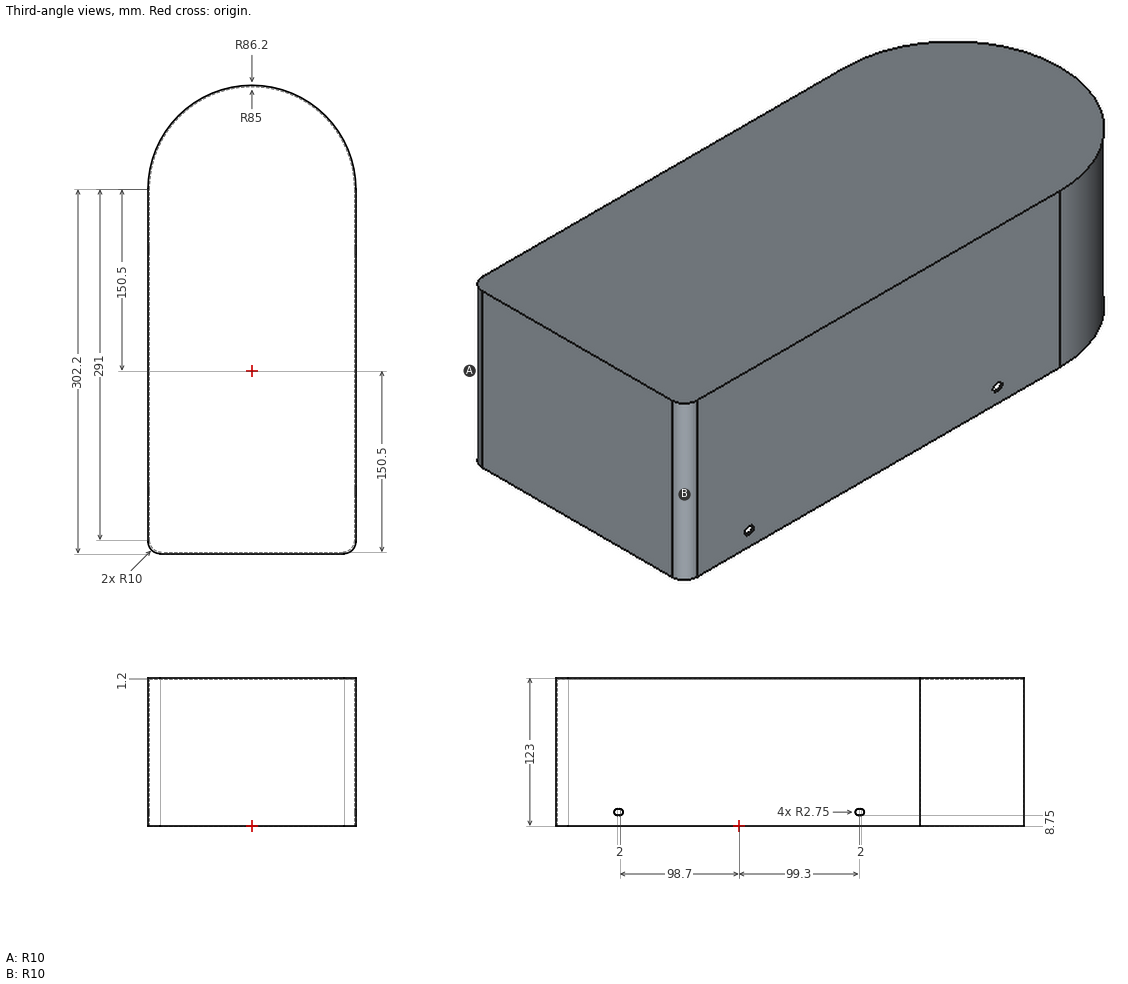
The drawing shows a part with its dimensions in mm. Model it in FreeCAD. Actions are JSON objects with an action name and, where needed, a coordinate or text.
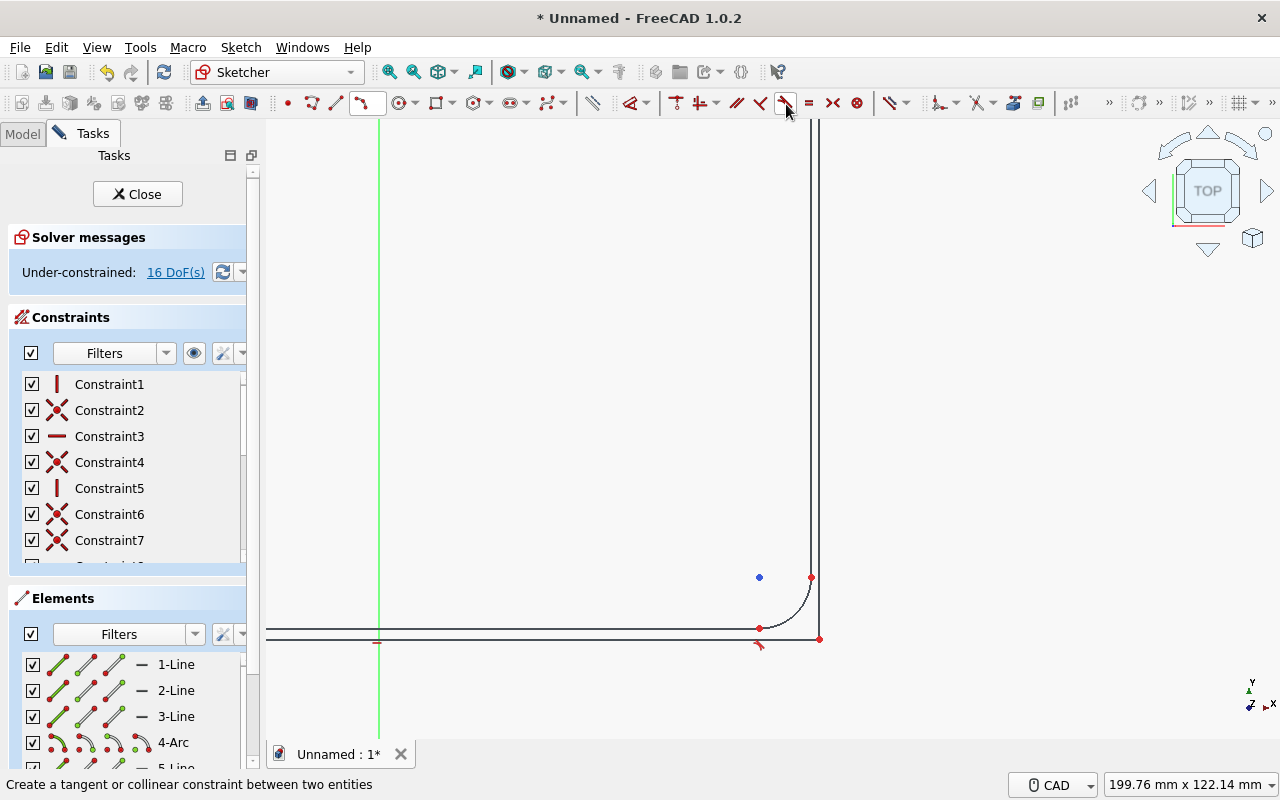
{"action": "scroll", "coordinate": [787, 626], "scroll_direction": "down", "scroll_amount": 8}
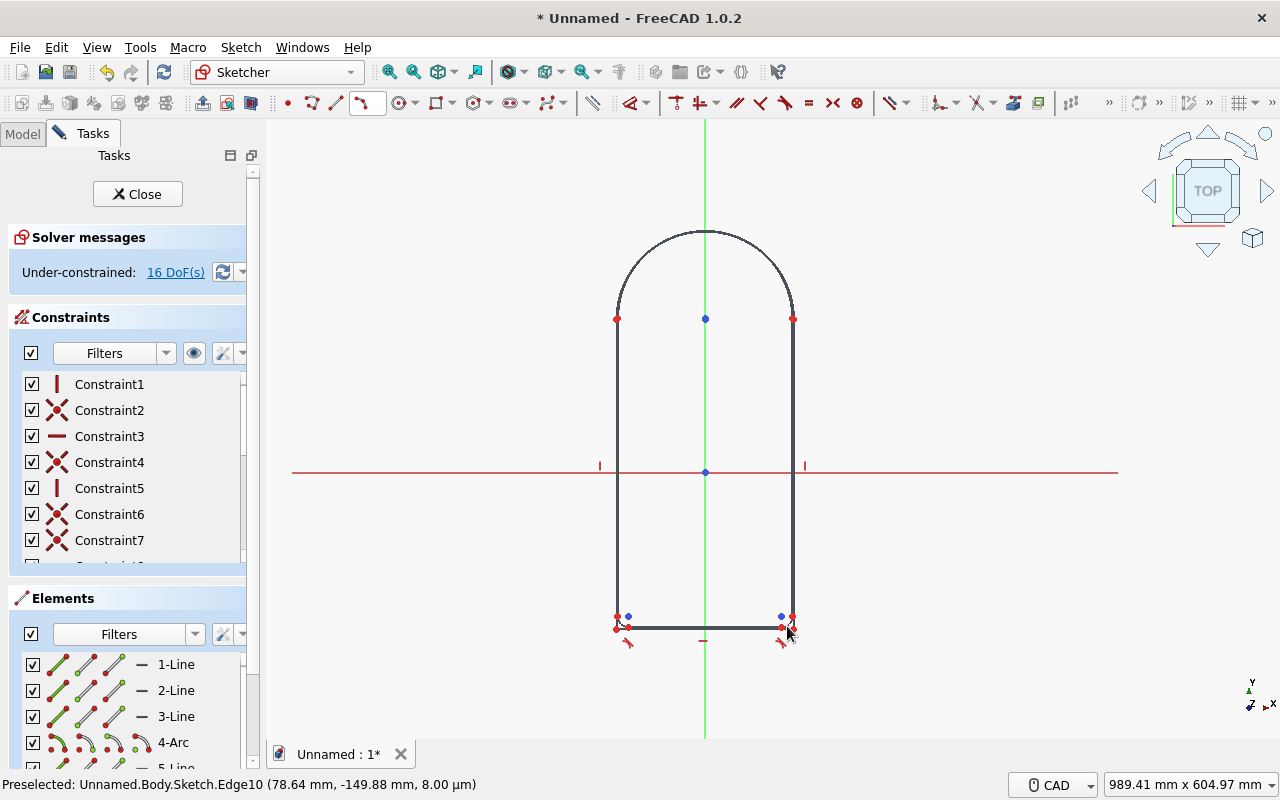
{"action": "scroll", "coordinate": [618, 527], "scroll_direction": "up", "scroll_amount": 12}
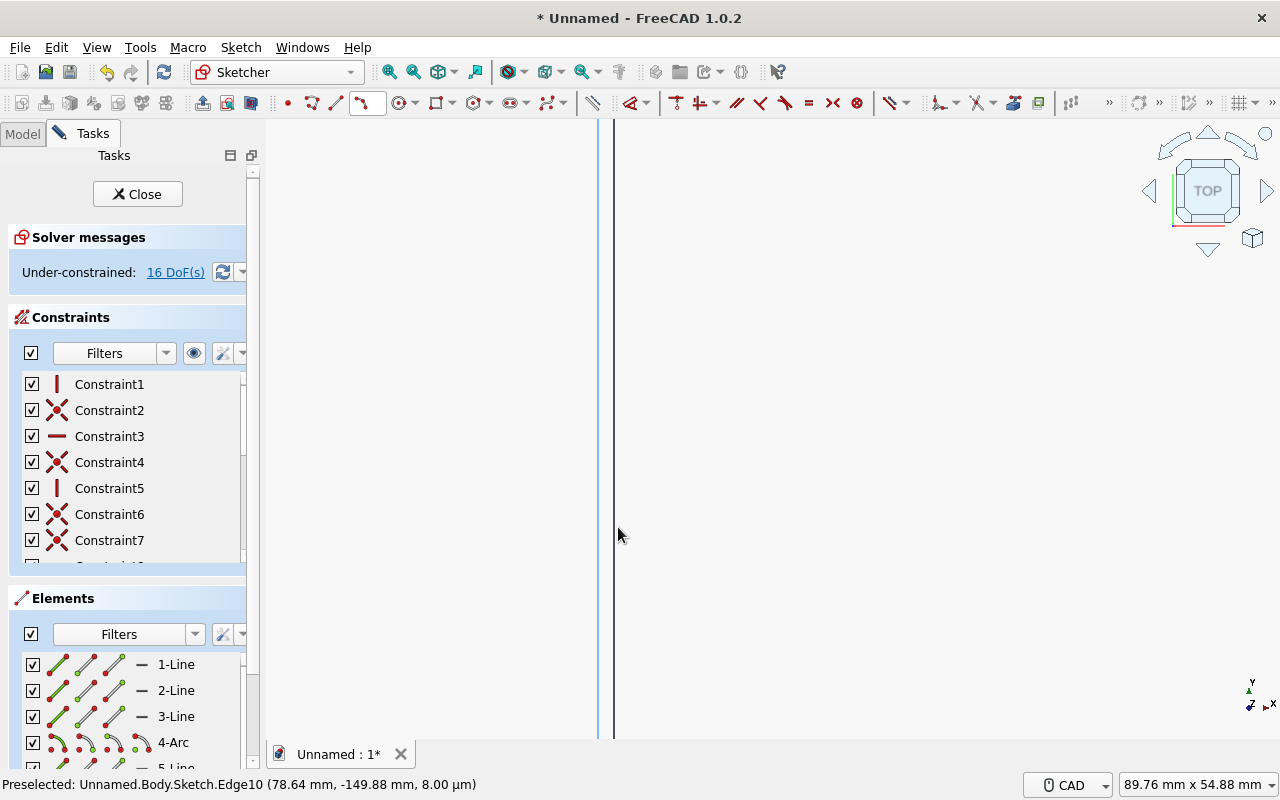
{"action": "left_click", "coordinate": [614, 525]}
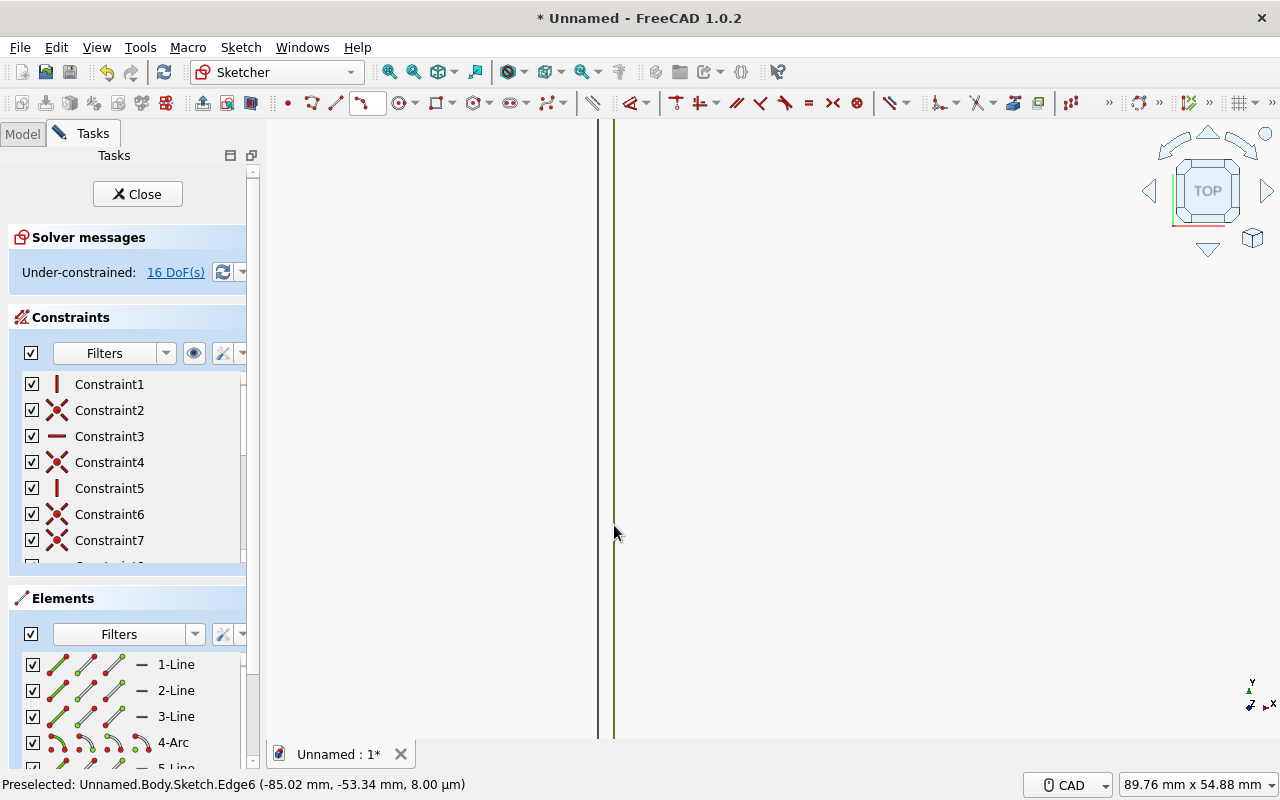
{"action": "scroll", "coordinate": [618, 527], "scroll_direction": "down", "scroll_amount": 12}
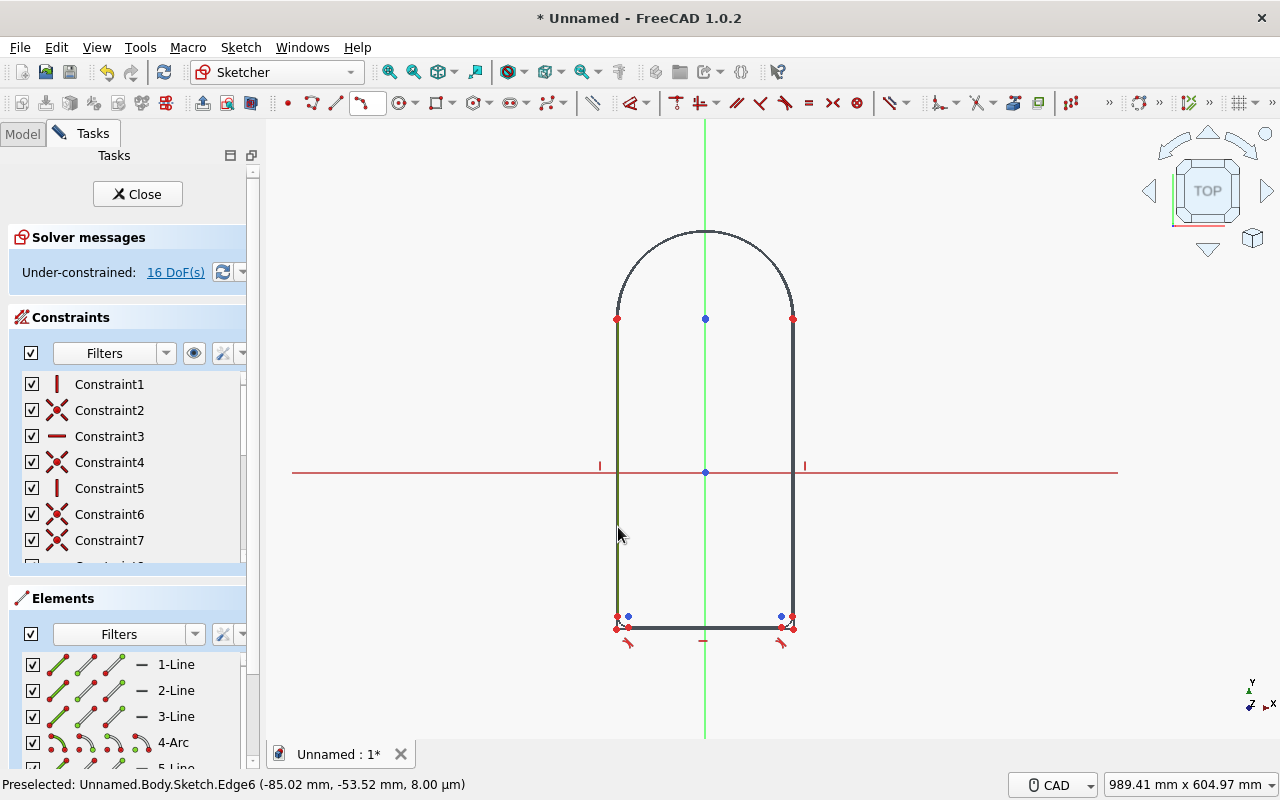
{"action": "scroll", "coordinate": [619, 622], "scroll_direction": "up", "scroll_amount": 9}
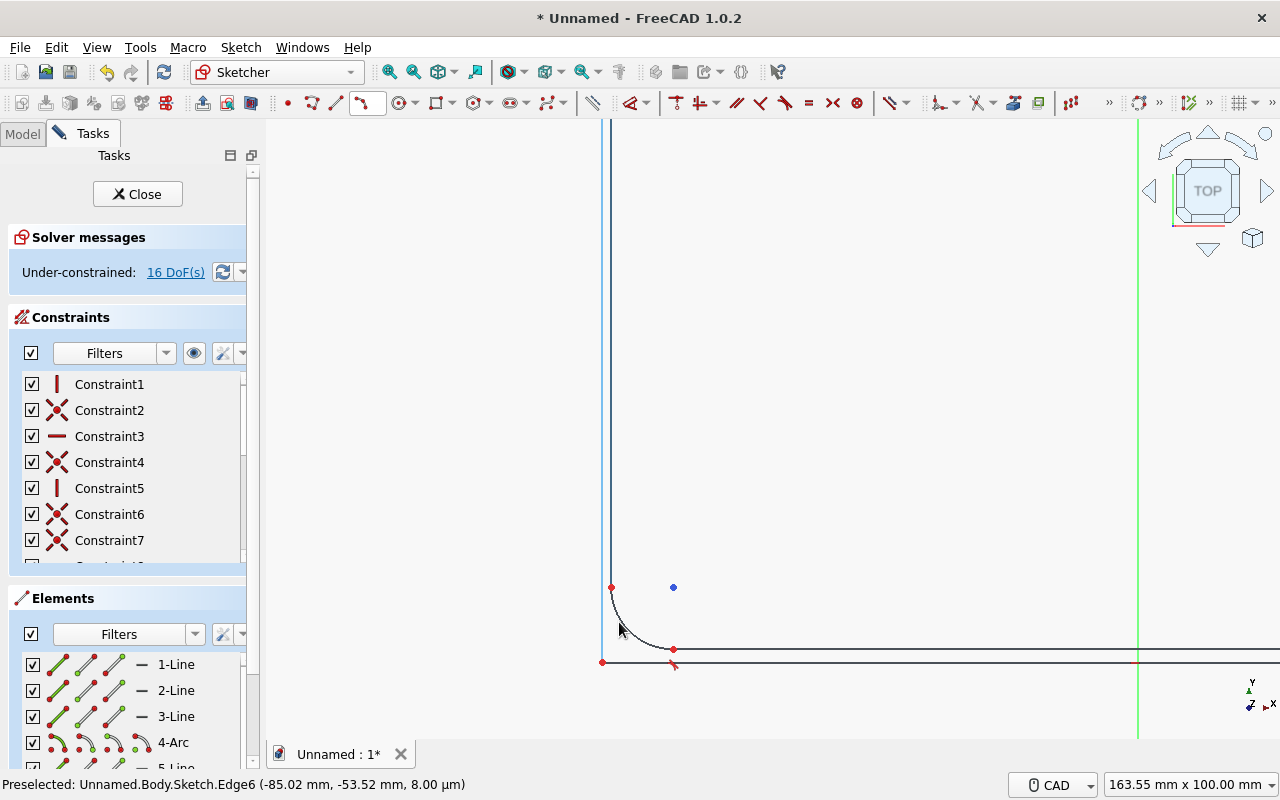
{"action": "left_click", "coordinate": [618, 615]}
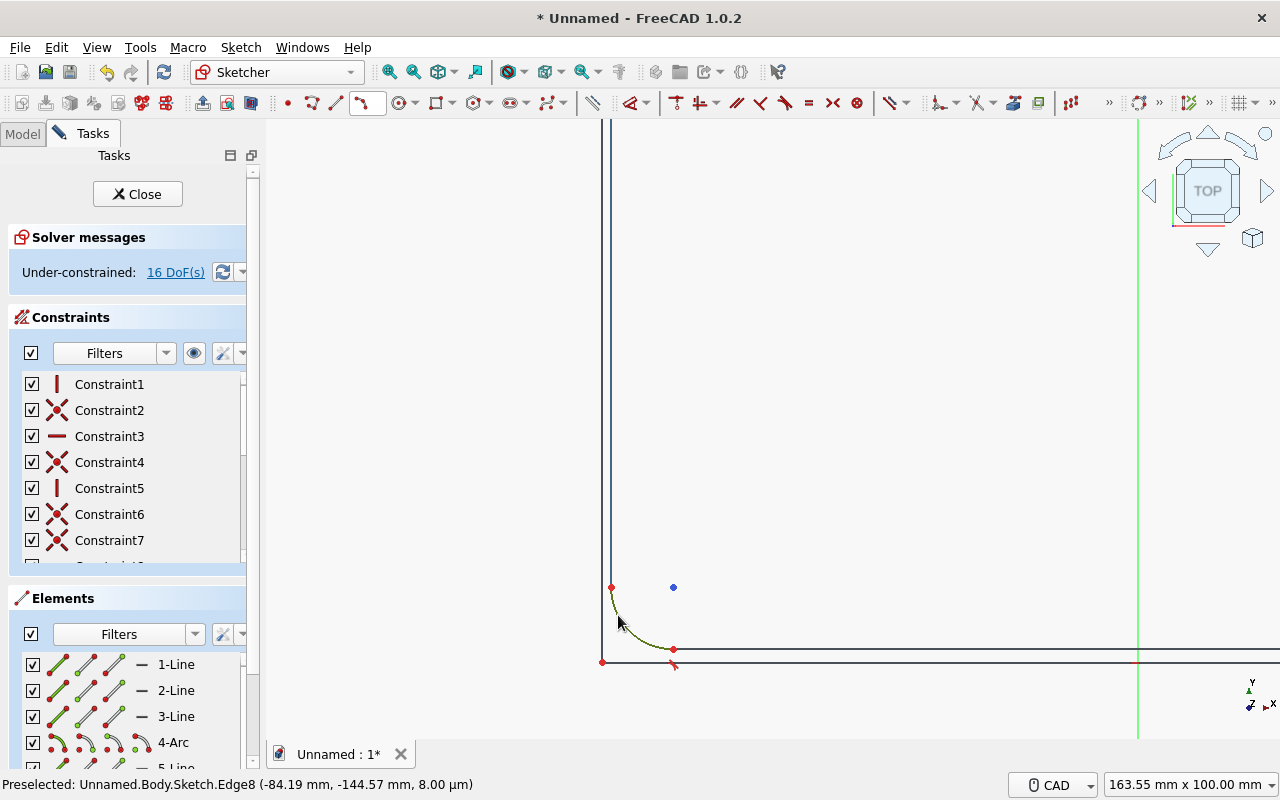
{"action": "key", "text": "t"}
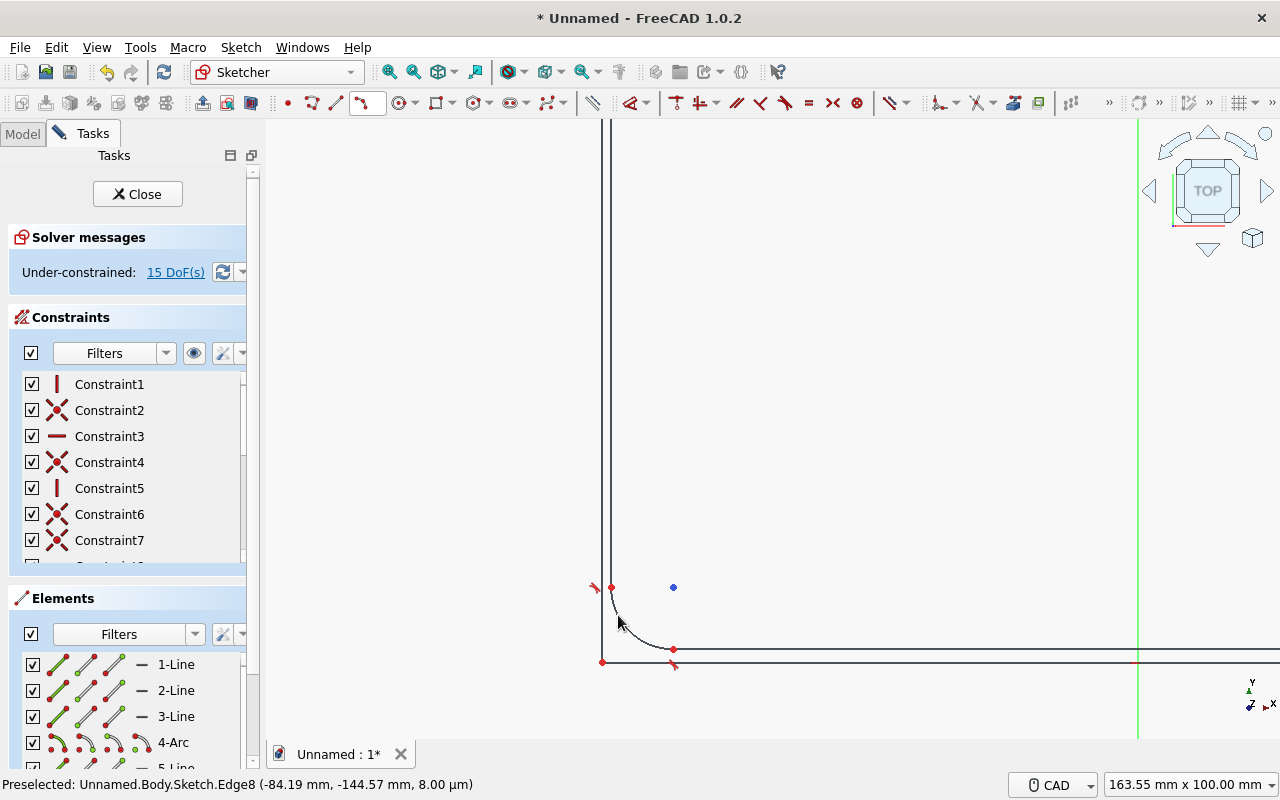
{"action": "scroll", "coordinate": [619, 622], "scroll_direction": "down", "scroll_amount": 9}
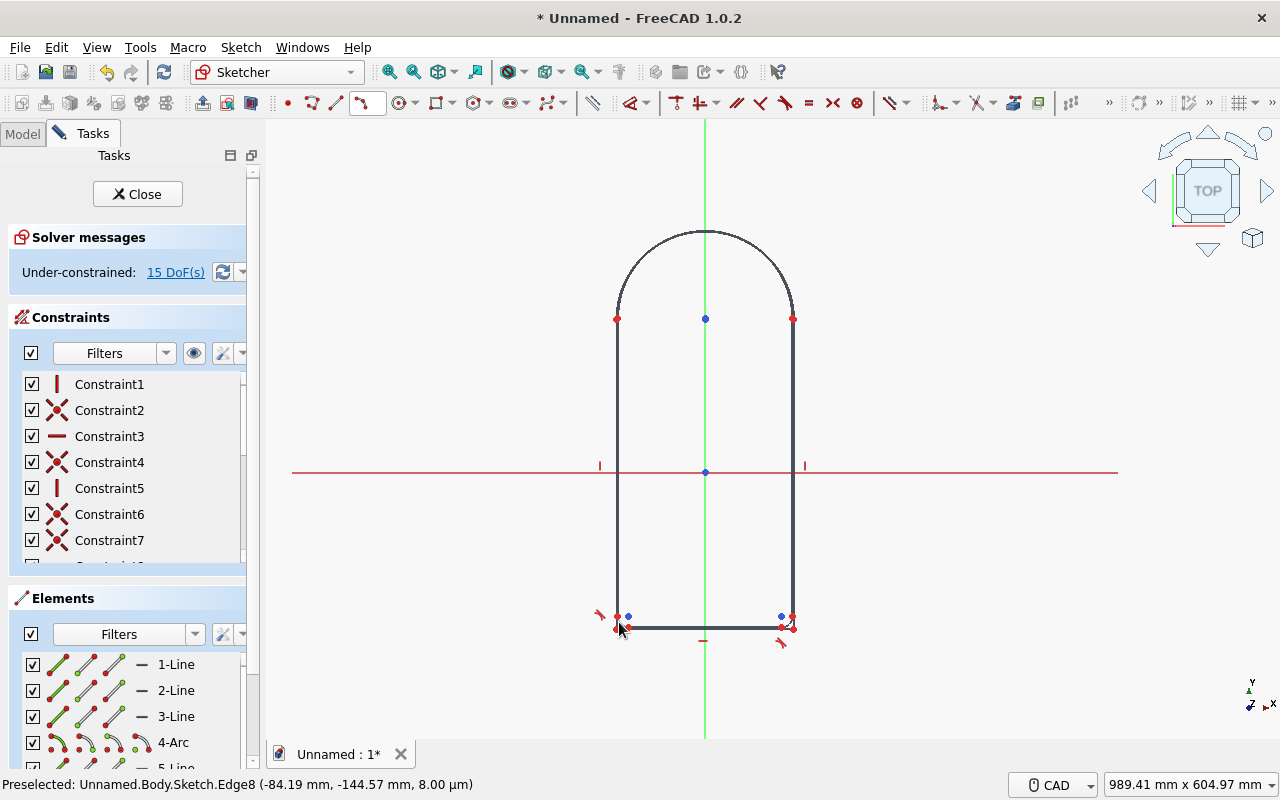
{"action": "scroll", "coordinate": [792, 408], "scroll_direction": "up", "scroll_amount": 11}